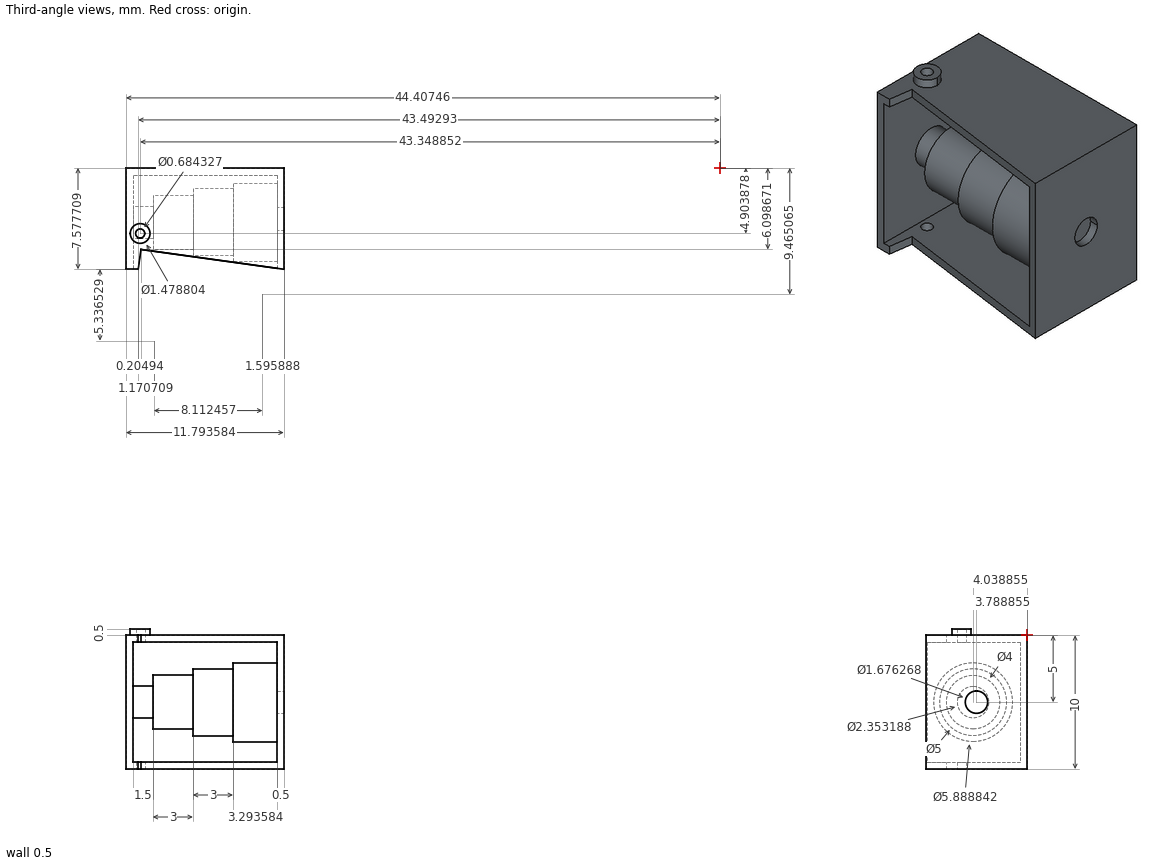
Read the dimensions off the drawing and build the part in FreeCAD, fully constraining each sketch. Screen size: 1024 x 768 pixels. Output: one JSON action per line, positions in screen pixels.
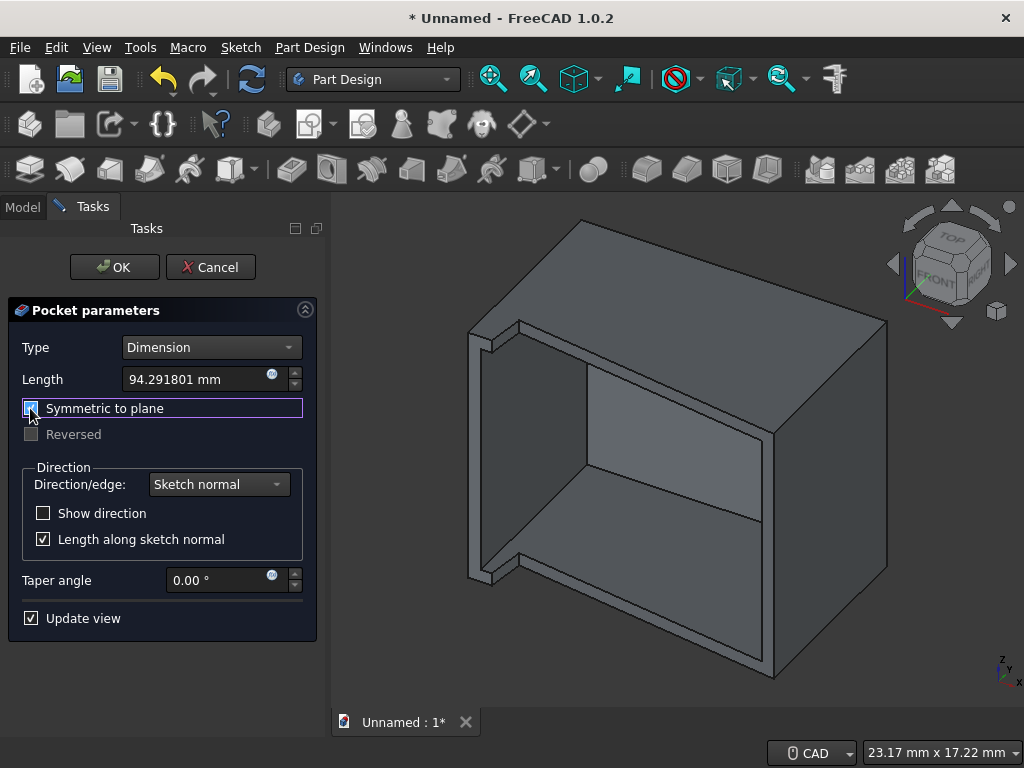
{"action": "left_click", "coordinate": [115, 267]}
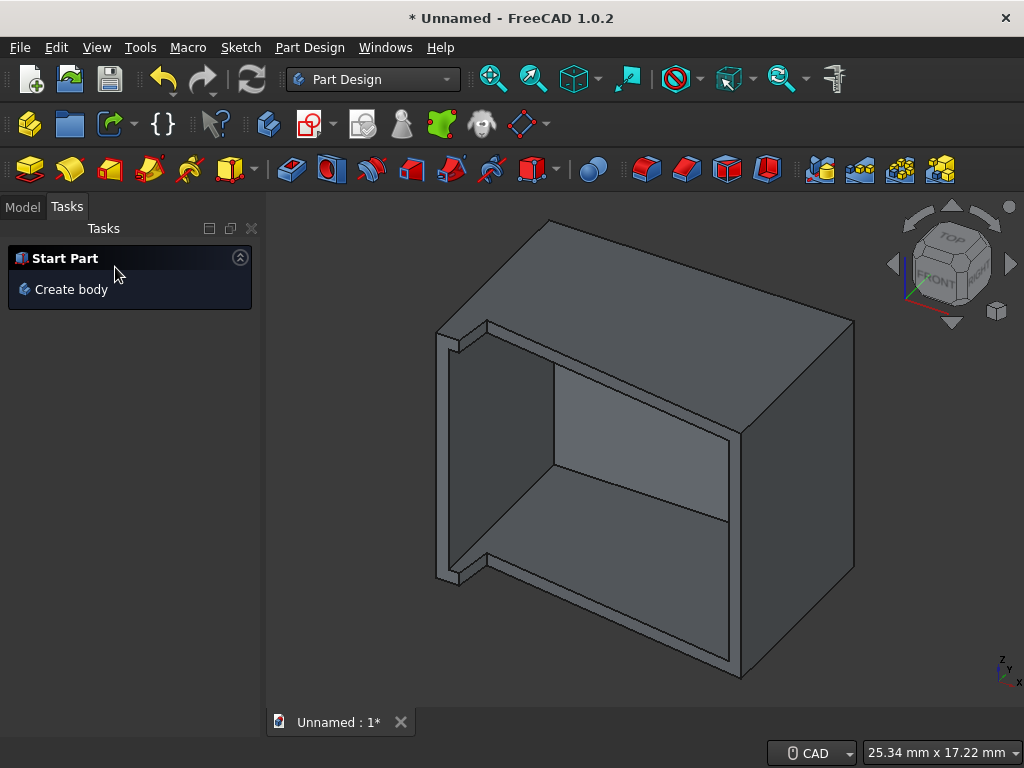
{"action": "left_click", "coordinate": [689, 340]}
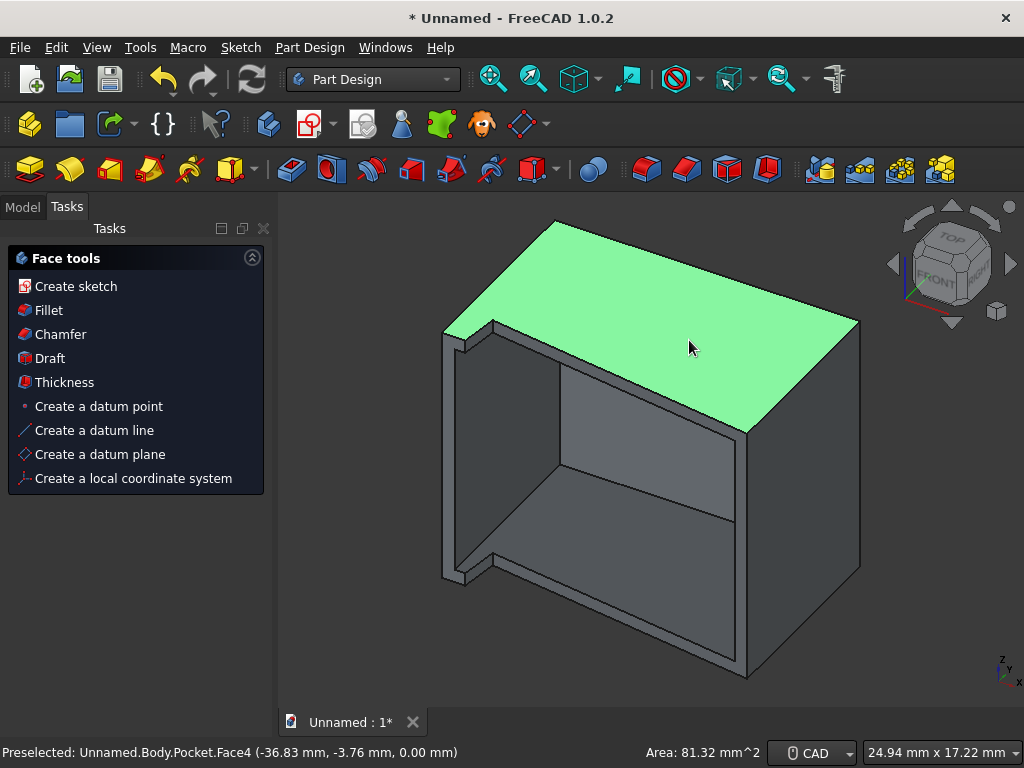
{"action": "left_click", "coordinate": [310, 124]}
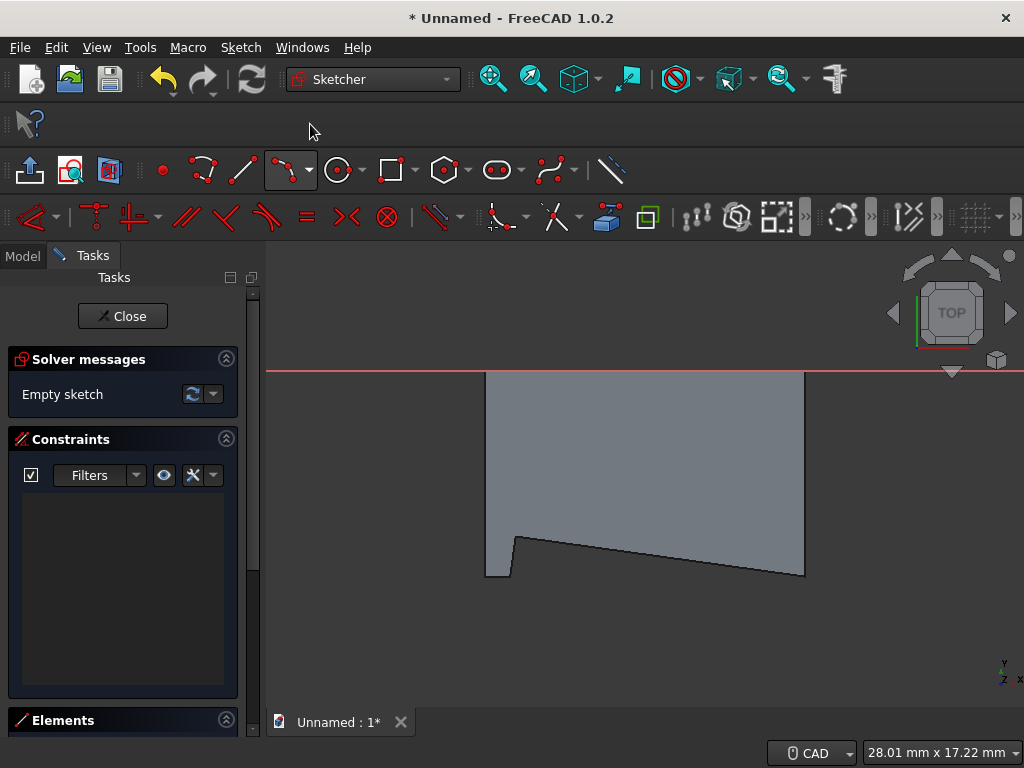
{"action": "scroll", "coordinate": [504, 509], "scroll_direction": "up", "scroll_amount": 10}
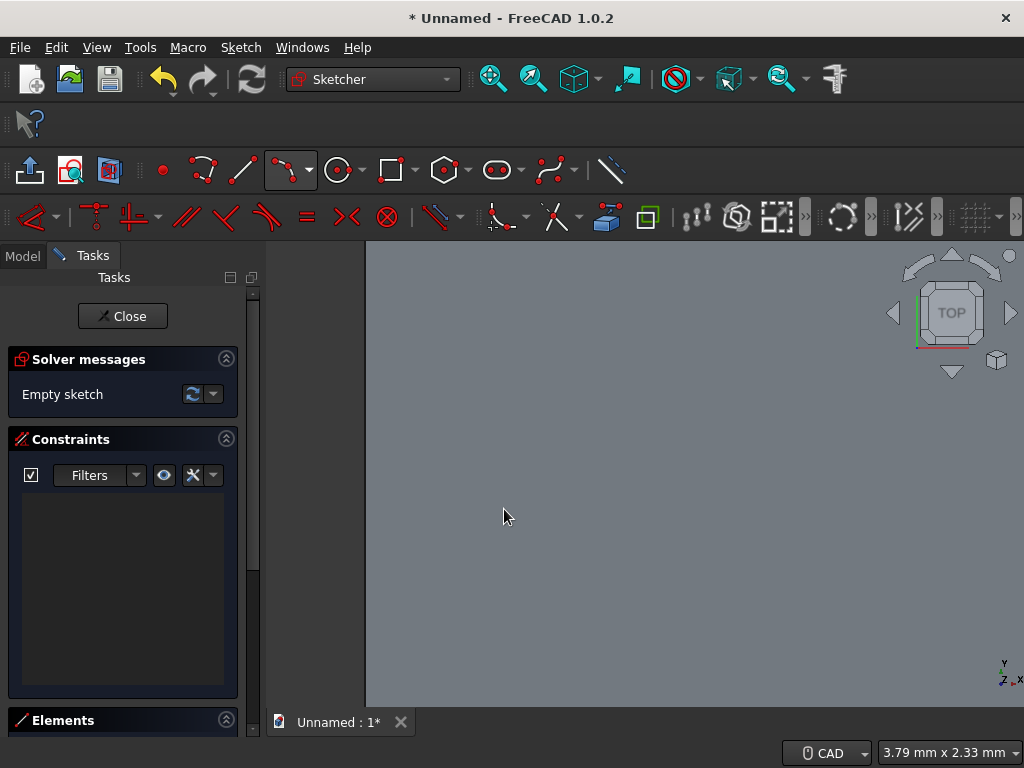
{"action": "left_click", "coordinate": [338, 170]}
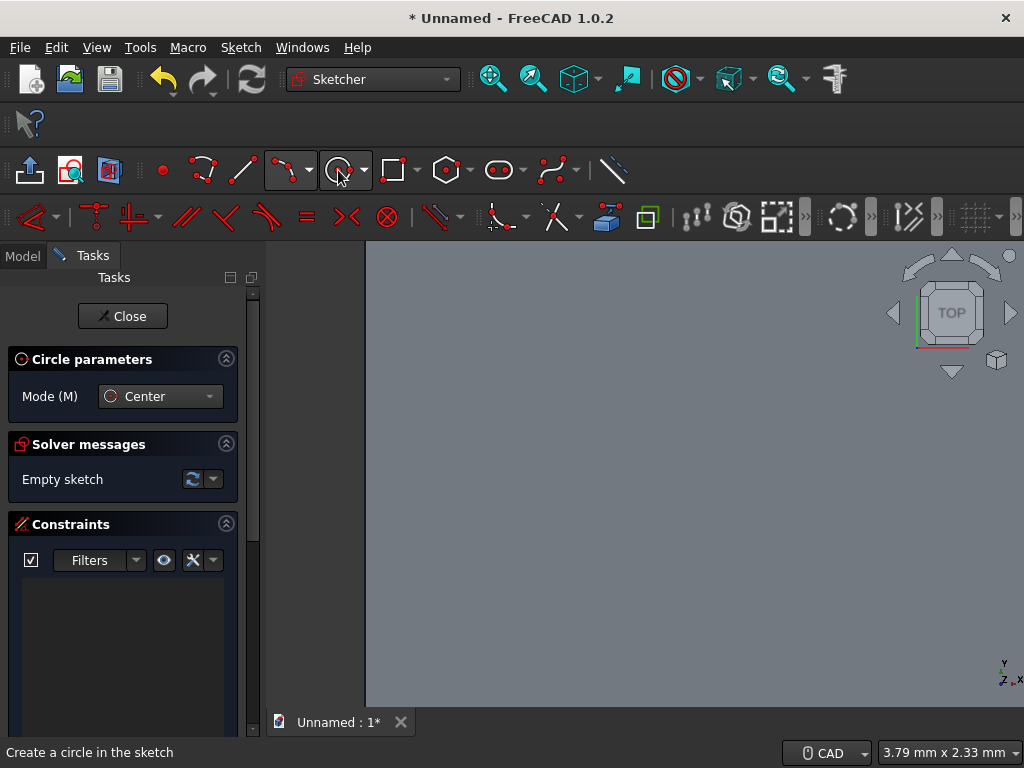
{"action": "left_click", "coordinate": [576, 470]}
{"action": "left_click", "coordinate": [681, 365]}
{"action": "key", "text": "Escape"}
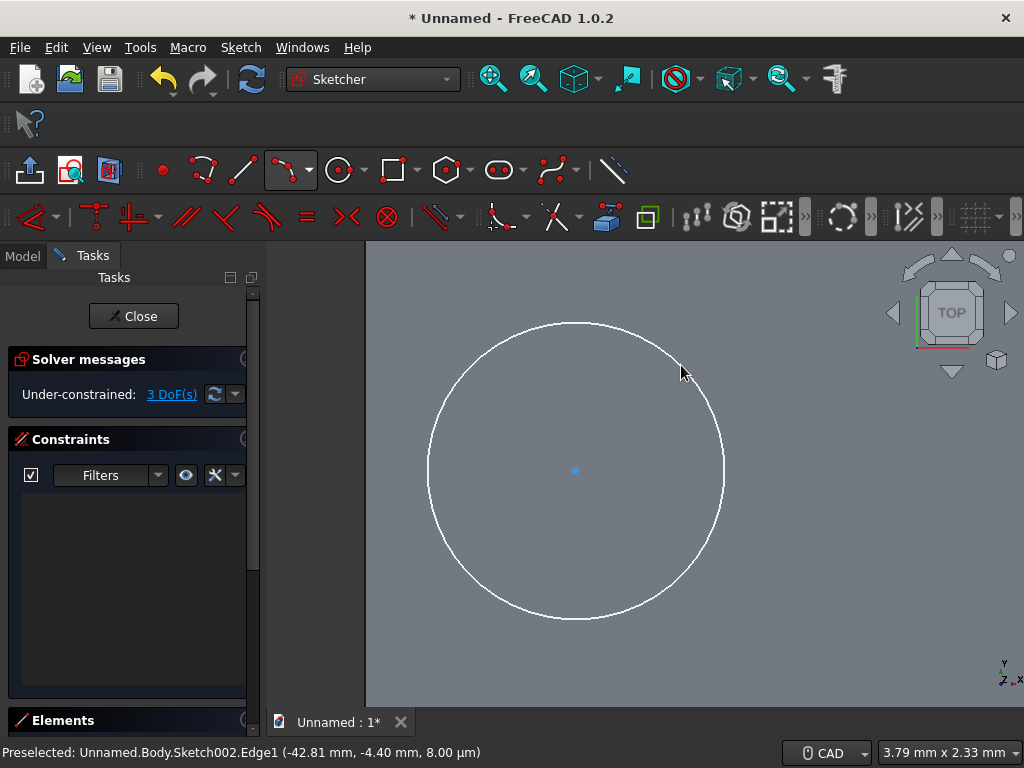
{"action": "left_click", "coordinate": [32, 218]}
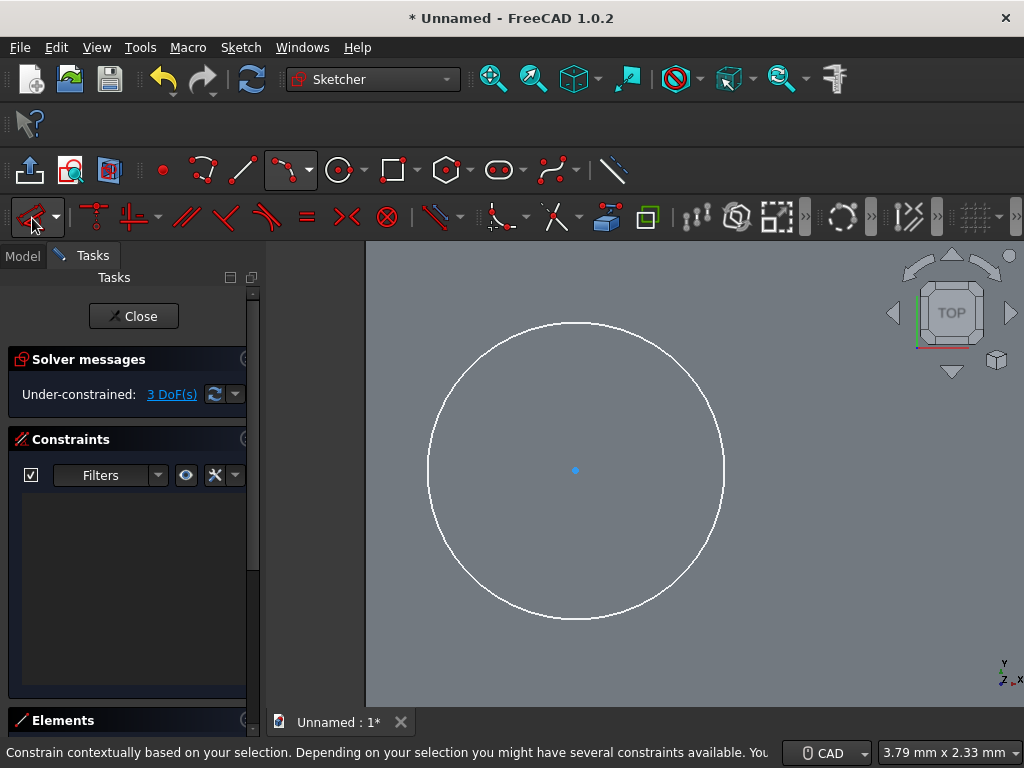
{"action": "left_click", "coordinate": [681, 366]}
{"action": "left_click", "coordinate": [704, 343]}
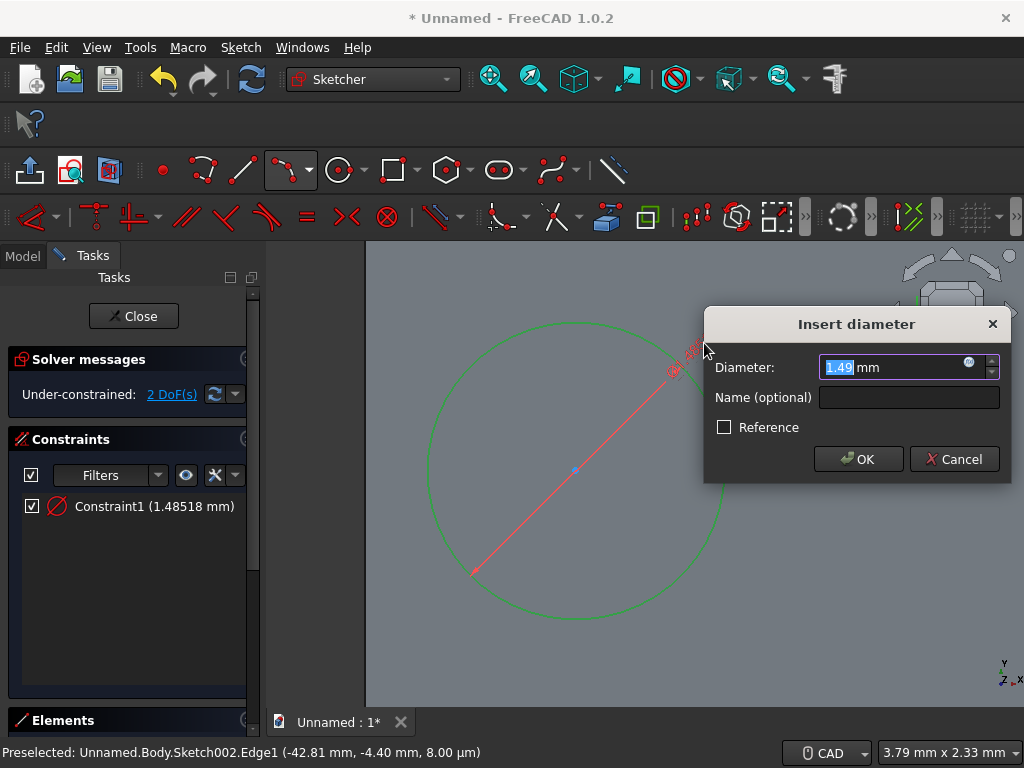
{"action": "type", "text": "1.478804"}
{"action": "key", "text": "Return"}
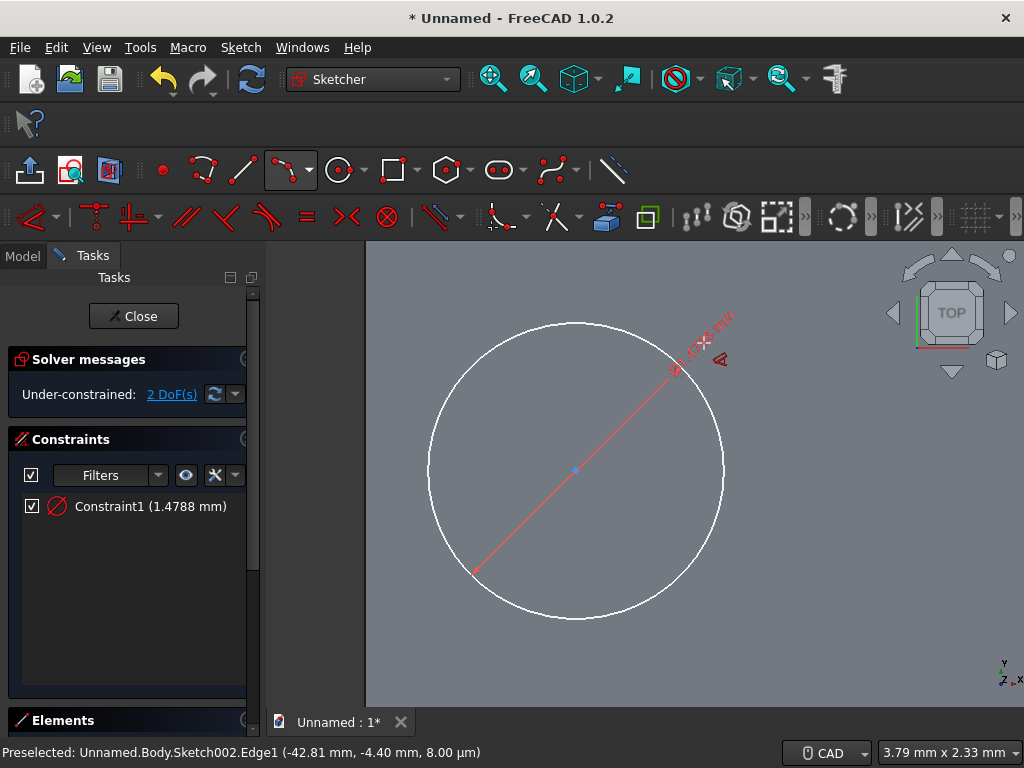
{"action": "left_click", "coordinate": [576, 471]}
{"action": "left_click", "coordinate": [542, 370]}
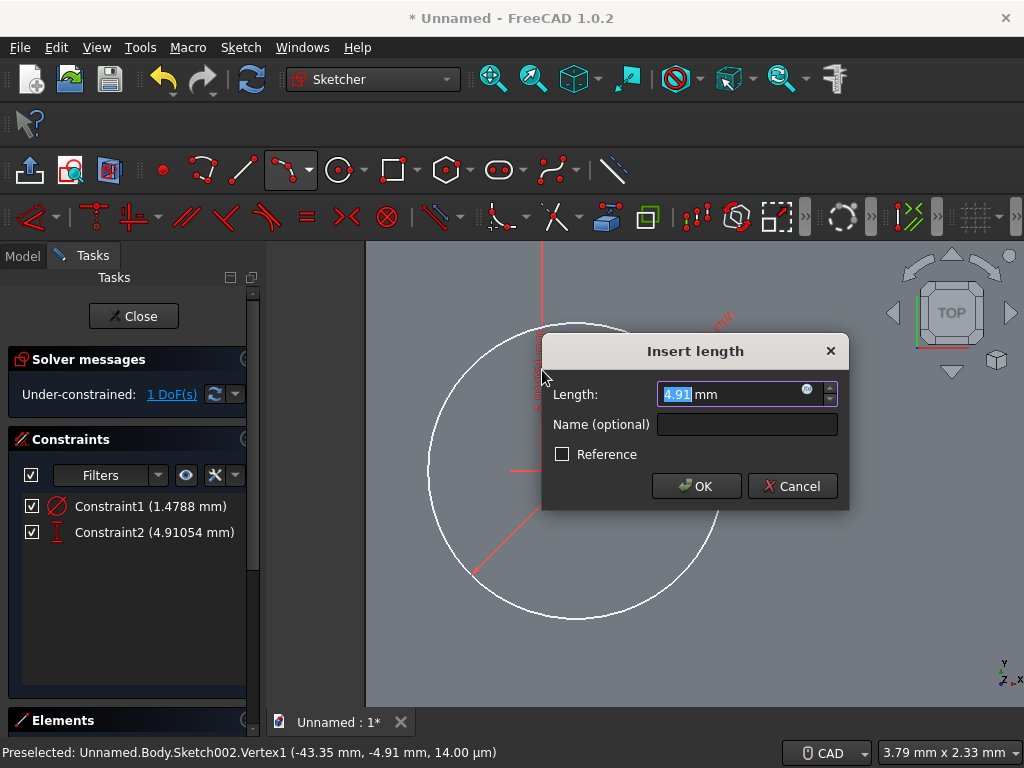
{"action": "type", "text": "4.903878"}
{"action": "key", "text": "Return"}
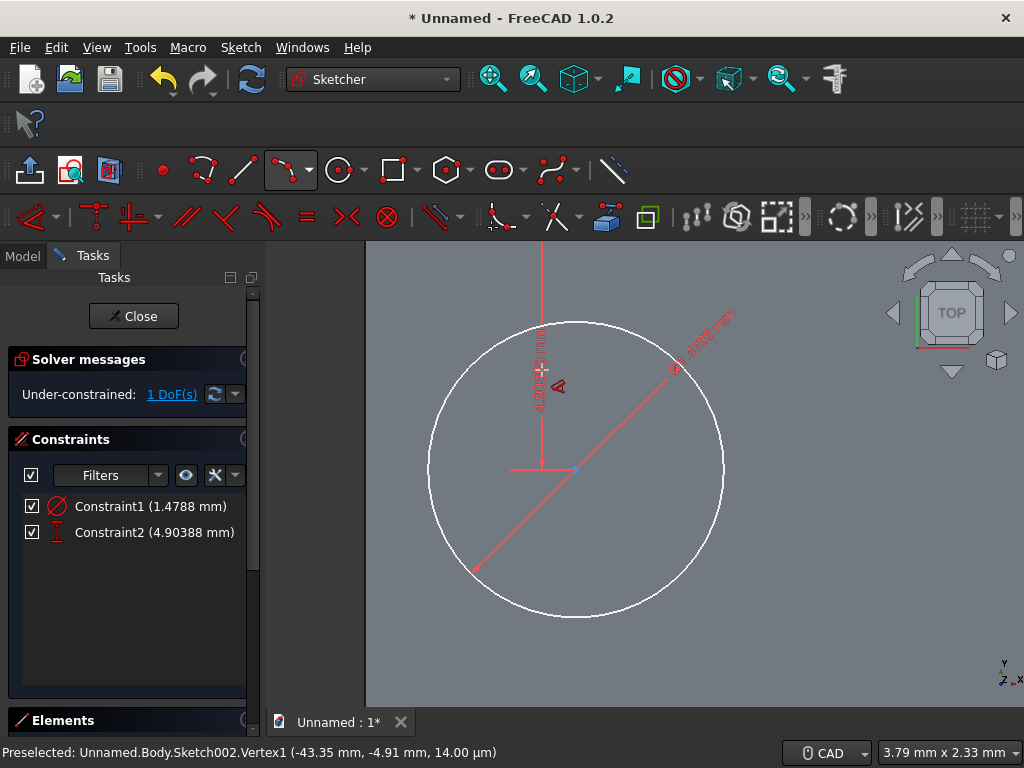
{"action": "left_click", "coordinate": [576, 470]}
{"action": "left_click", "coordinate": [652, 504]}